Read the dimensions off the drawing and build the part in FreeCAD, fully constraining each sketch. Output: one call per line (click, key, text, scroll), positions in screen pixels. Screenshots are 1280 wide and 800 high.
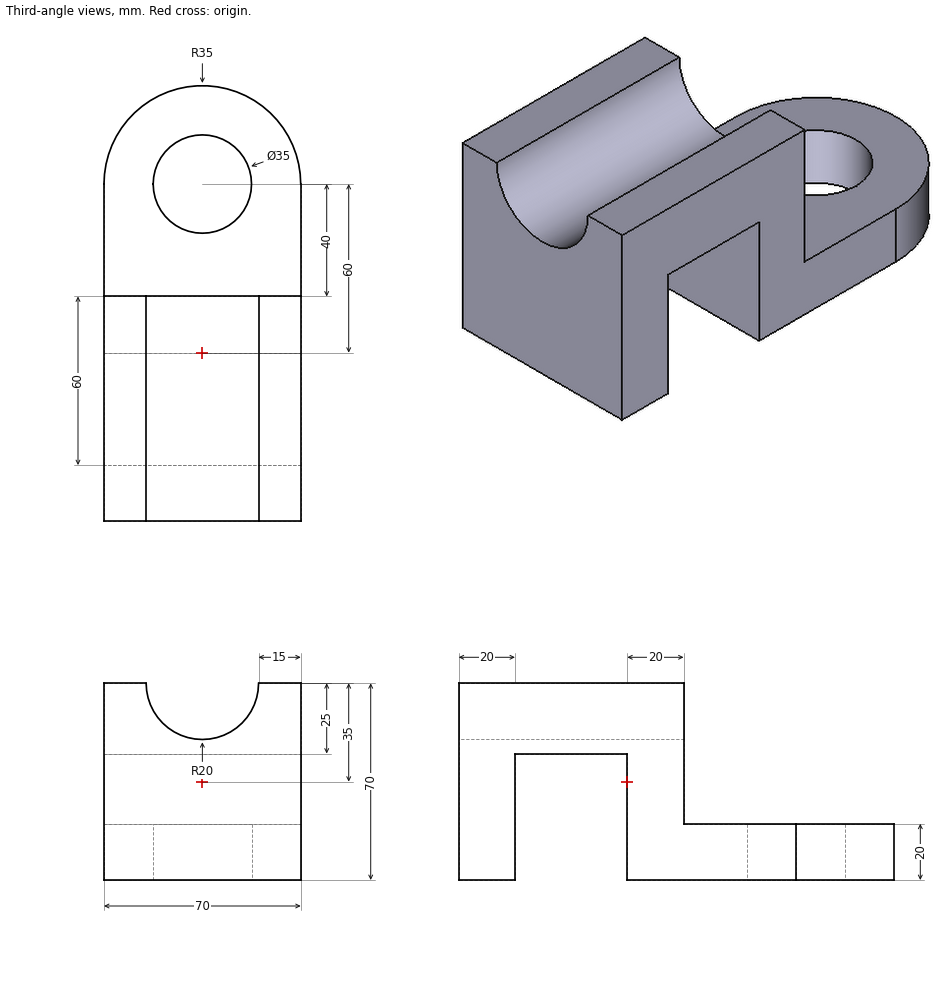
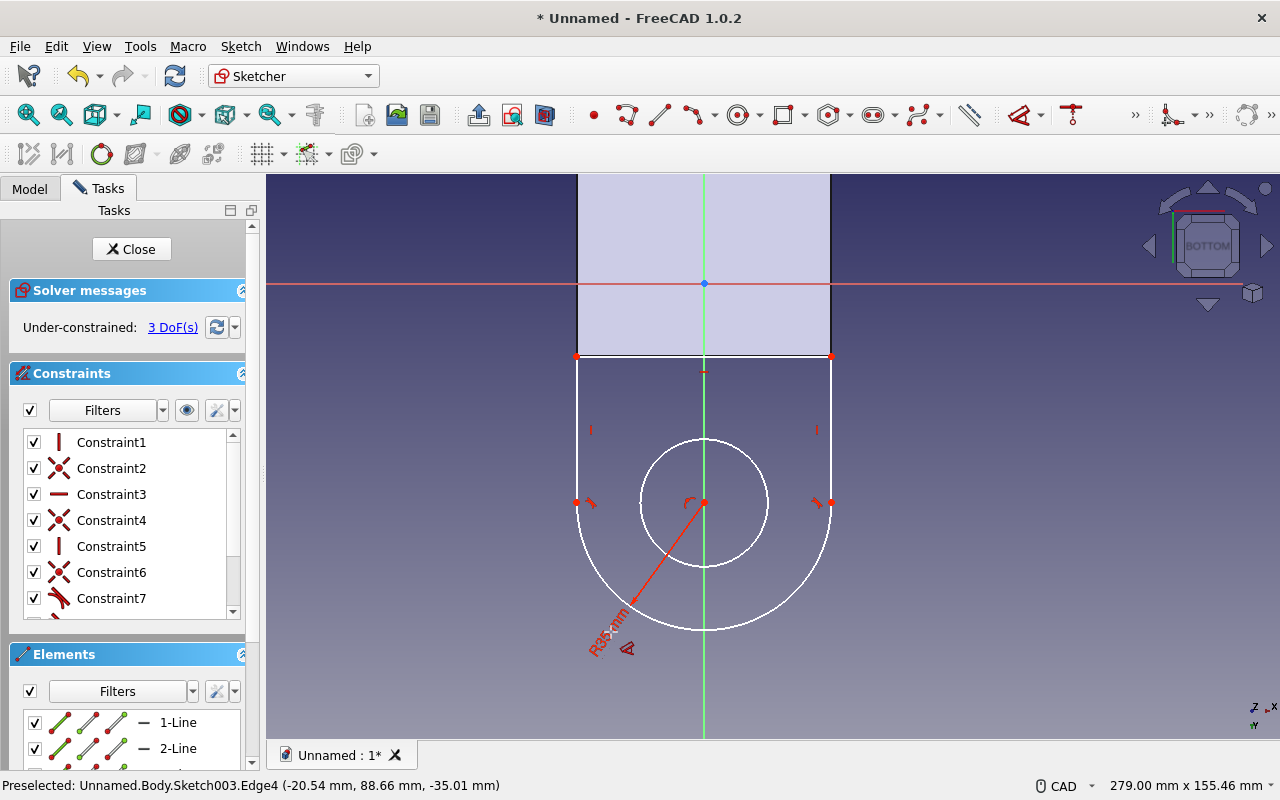
click(749, 458)
click(772, 435)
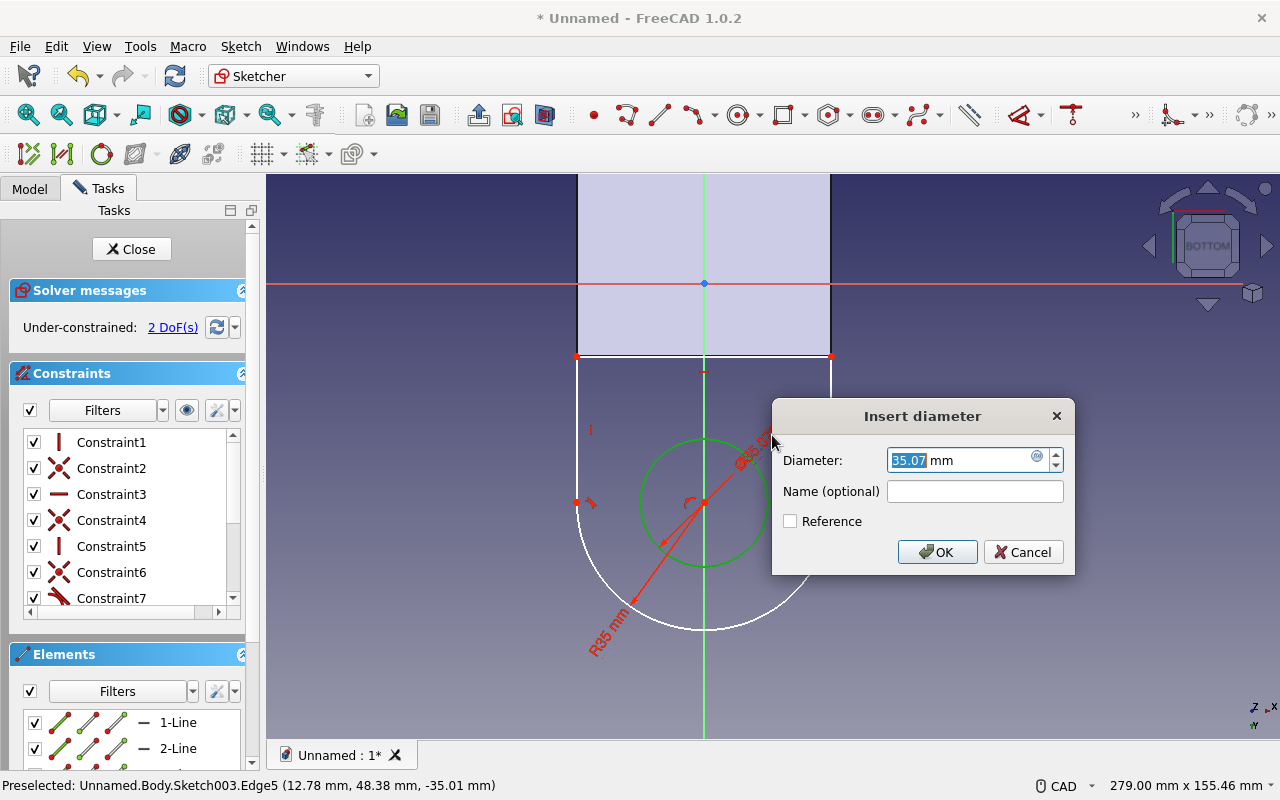
text(35)
key(Return)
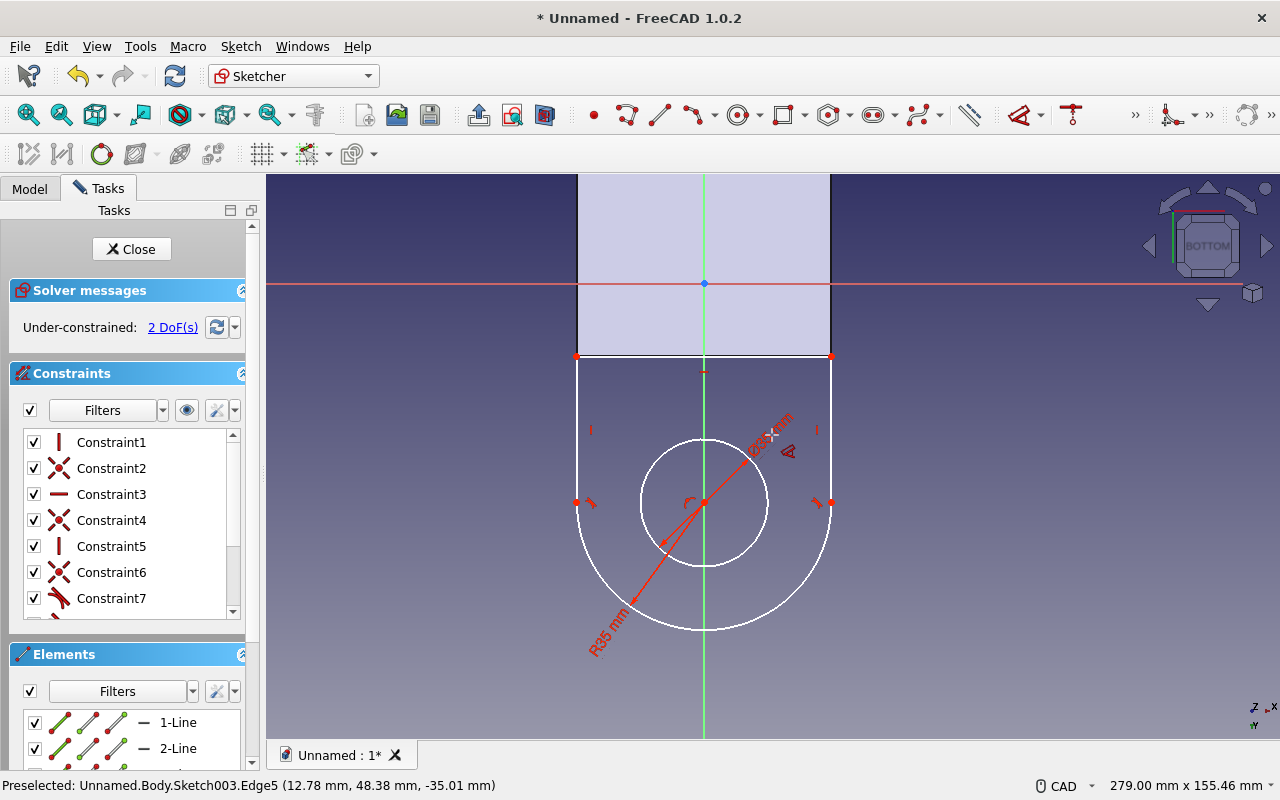
click(831, 459)
click(865, 430)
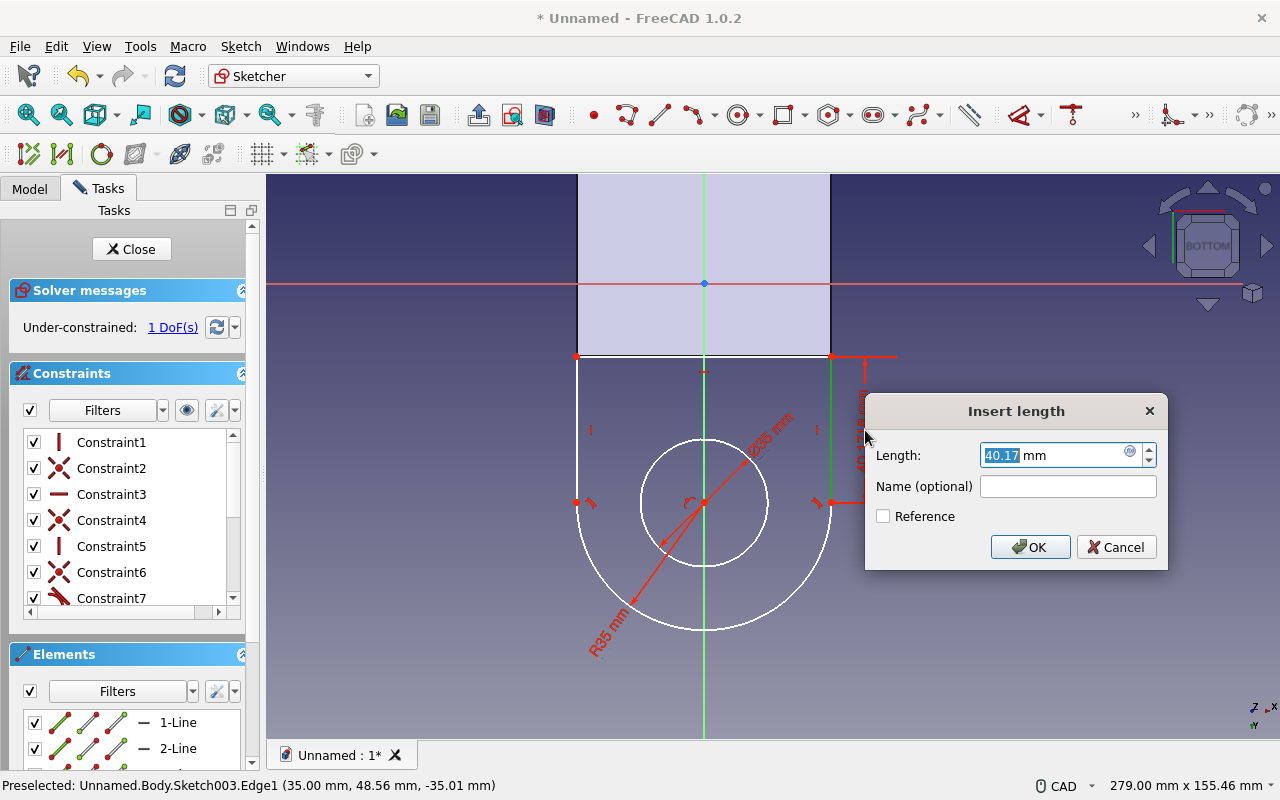
text(40)
key(Return)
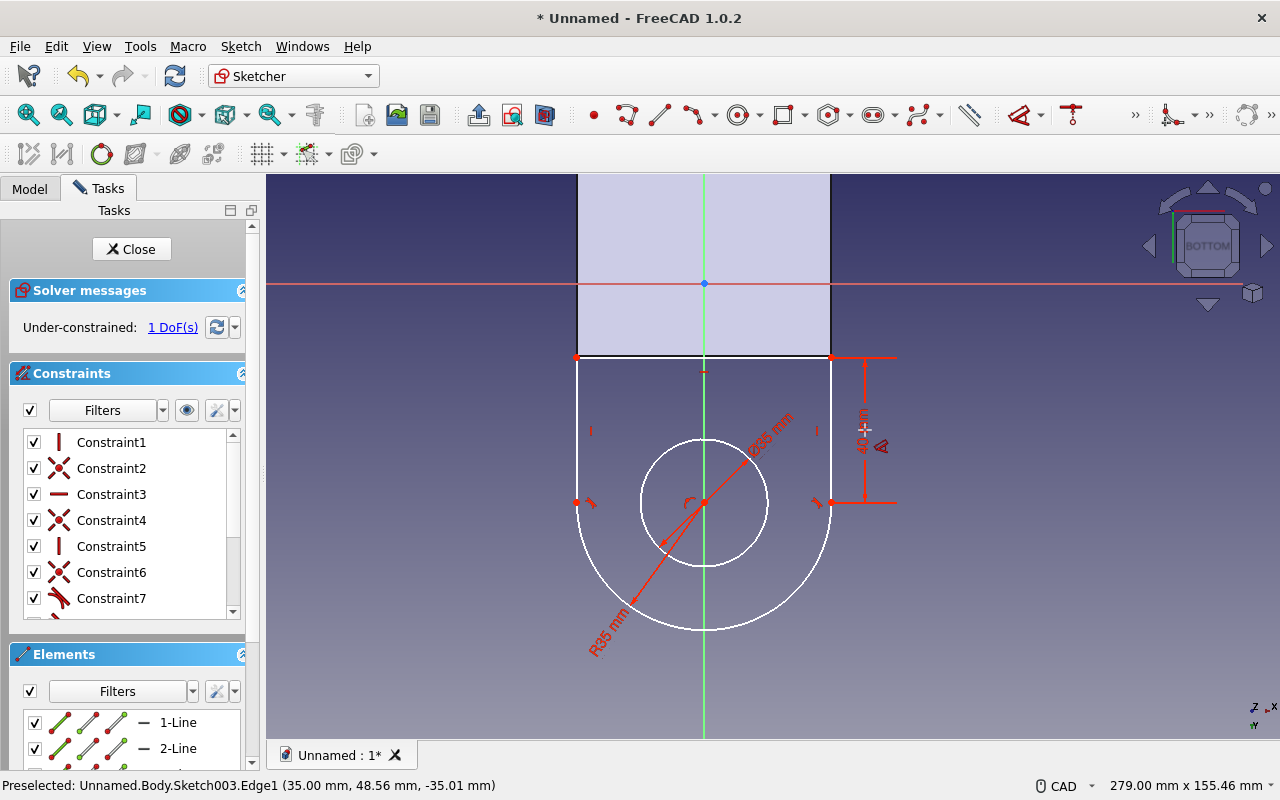
click(704, 503)
click(738, 393)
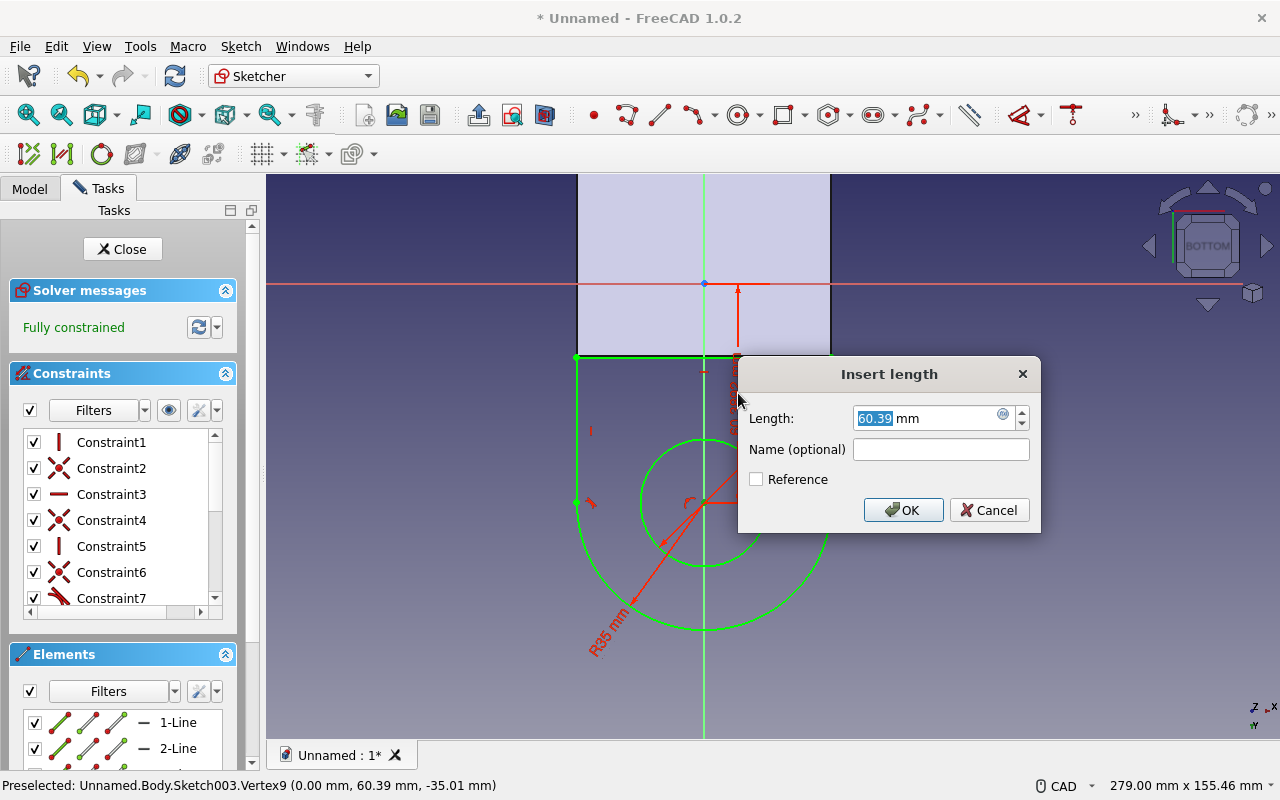
text(60)
key(Return)
key(Escape)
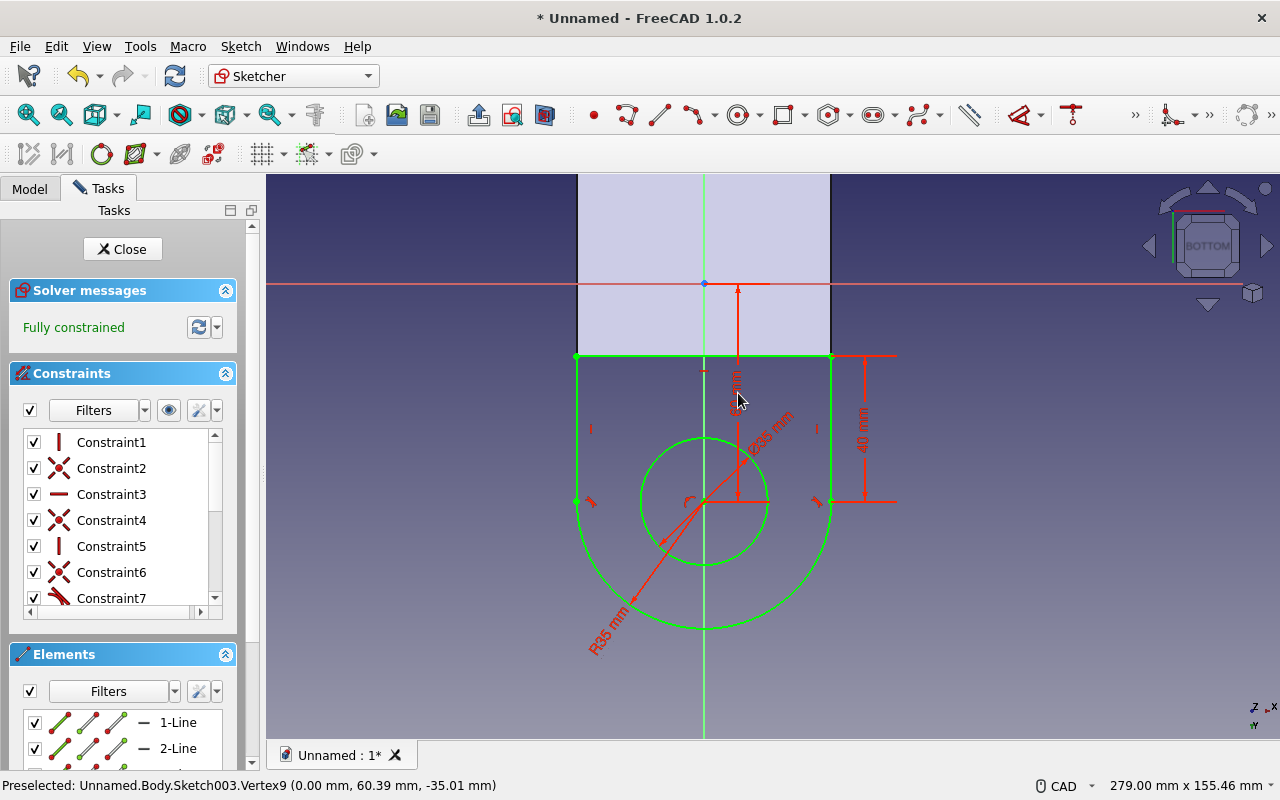
click(123, 249)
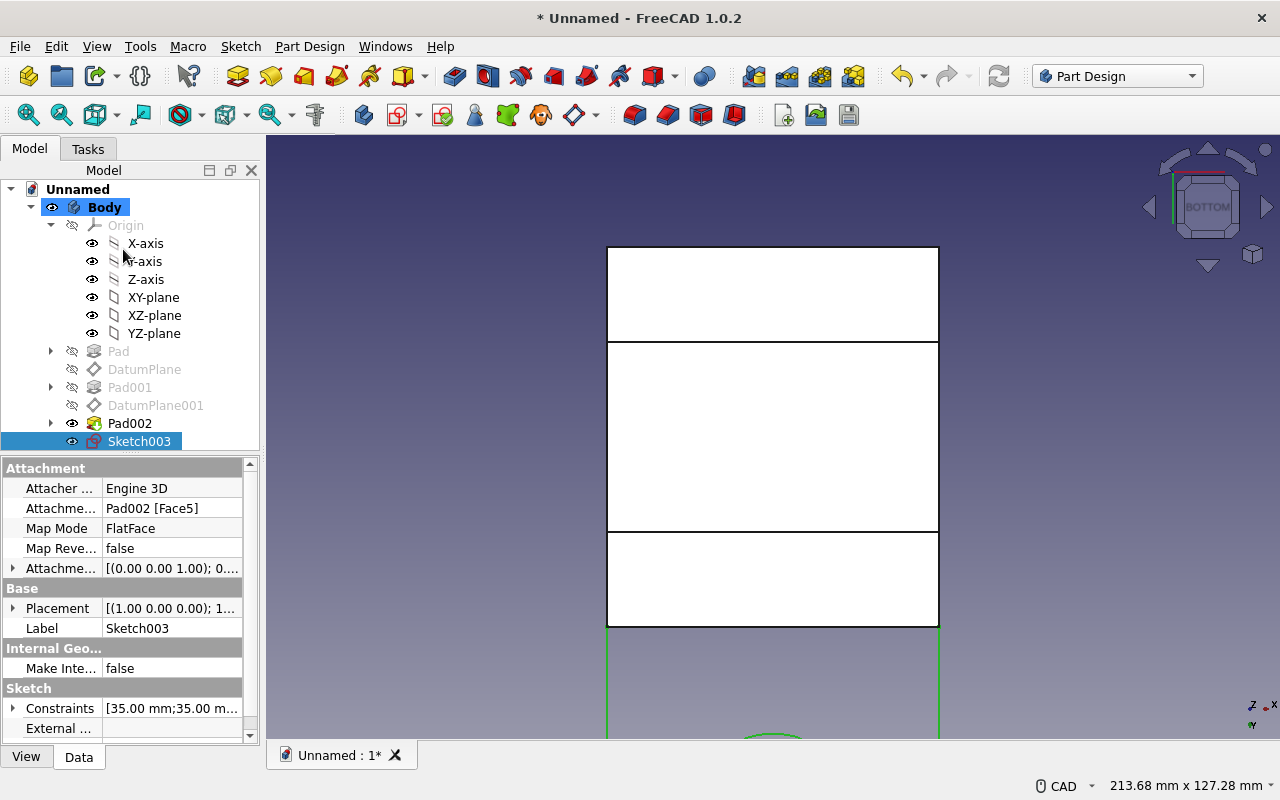
click(238, 76)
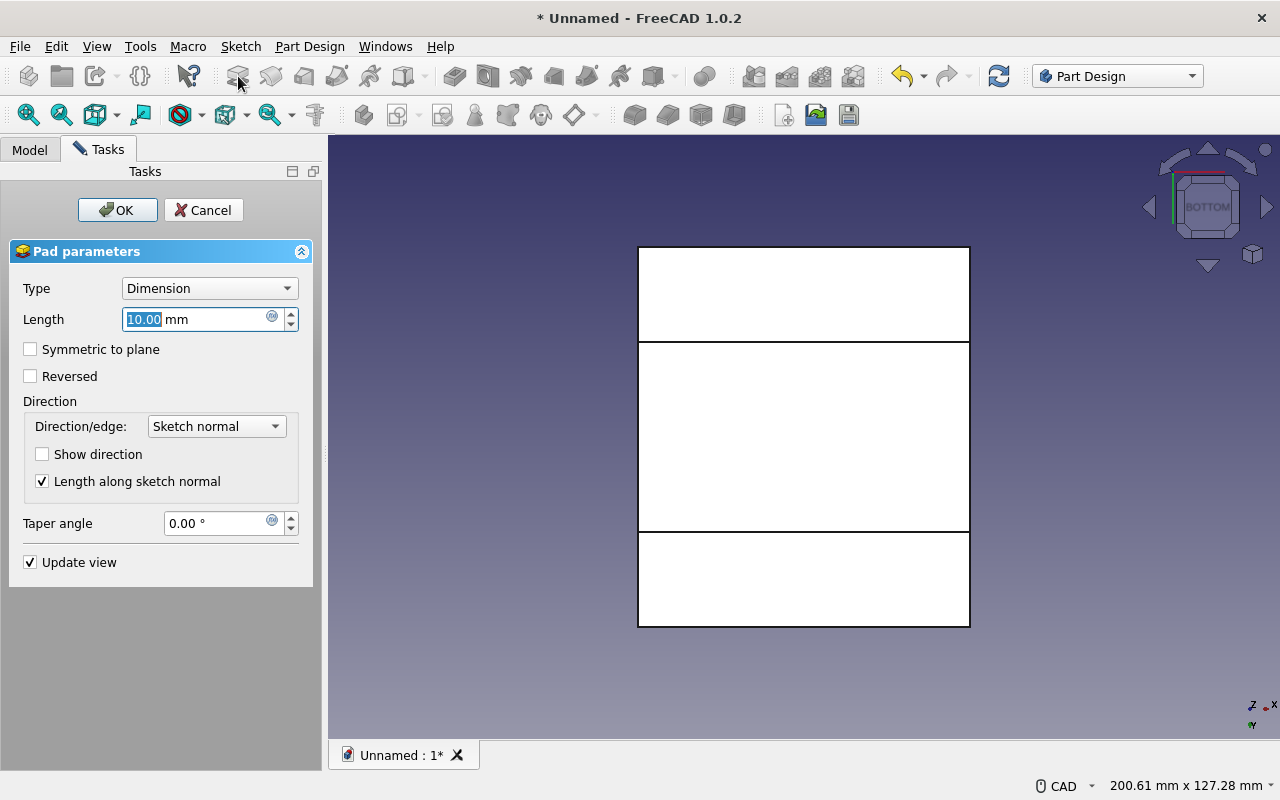
text(20)
key(Tab)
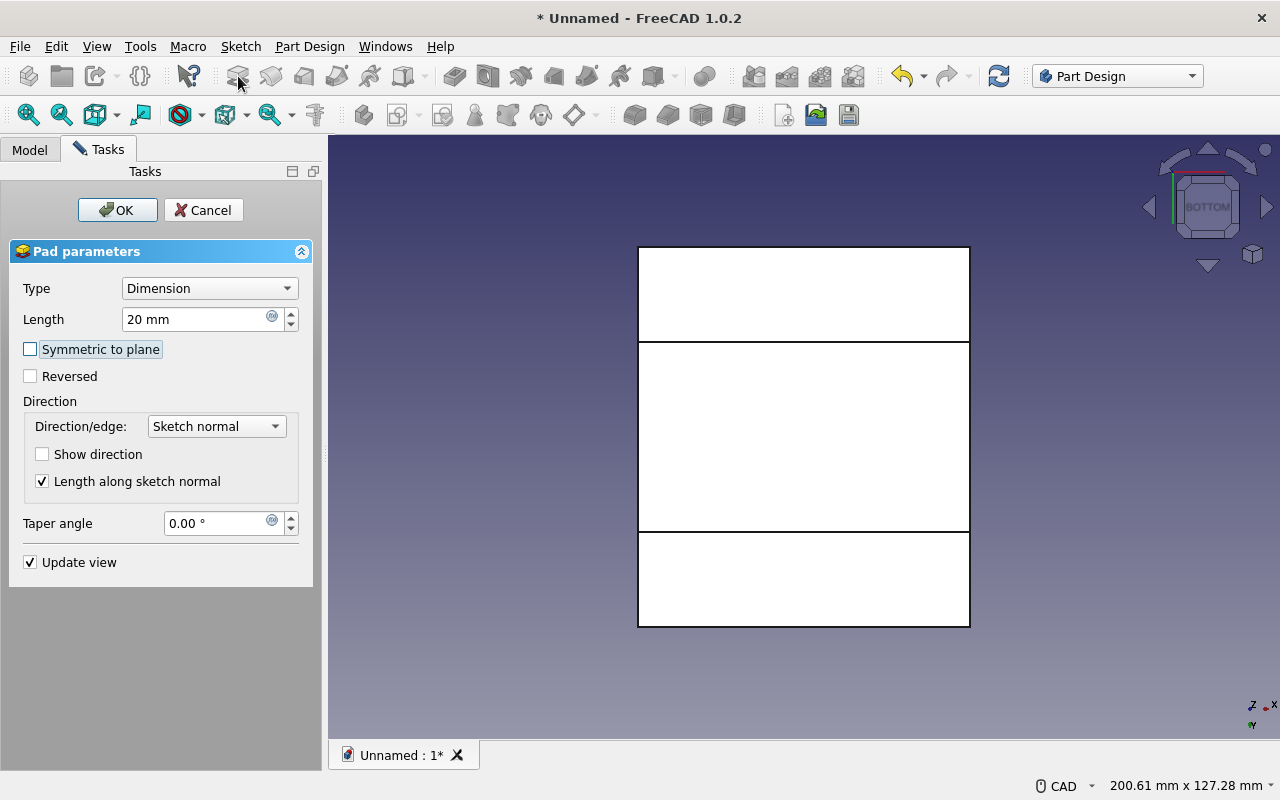
click(31, 376)